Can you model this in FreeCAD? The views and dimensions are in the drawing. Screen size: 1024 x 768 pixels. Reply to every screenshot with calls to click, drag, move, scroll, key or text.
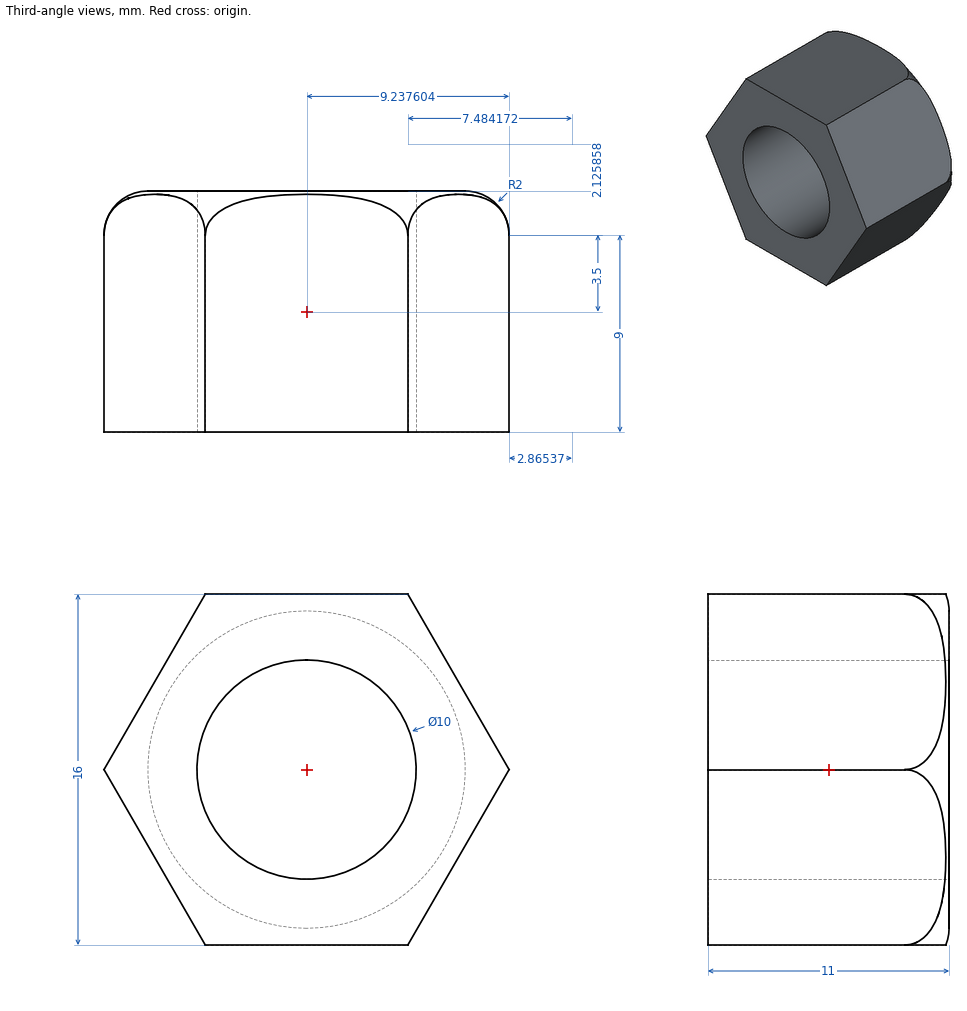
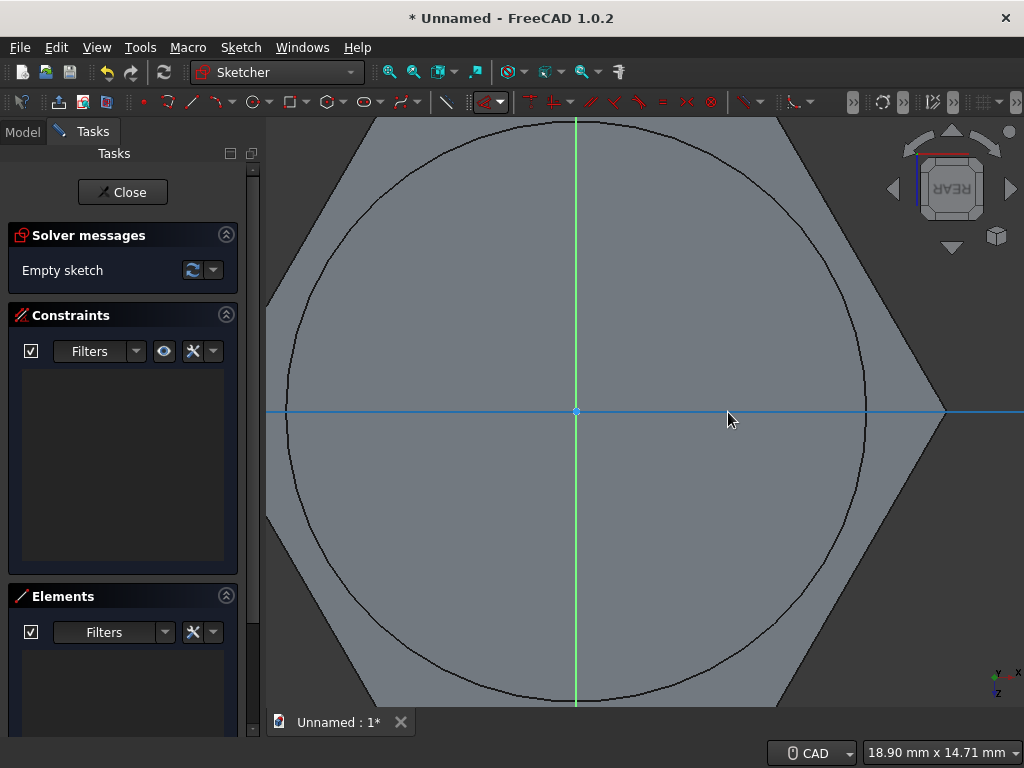
key(g)
key(c)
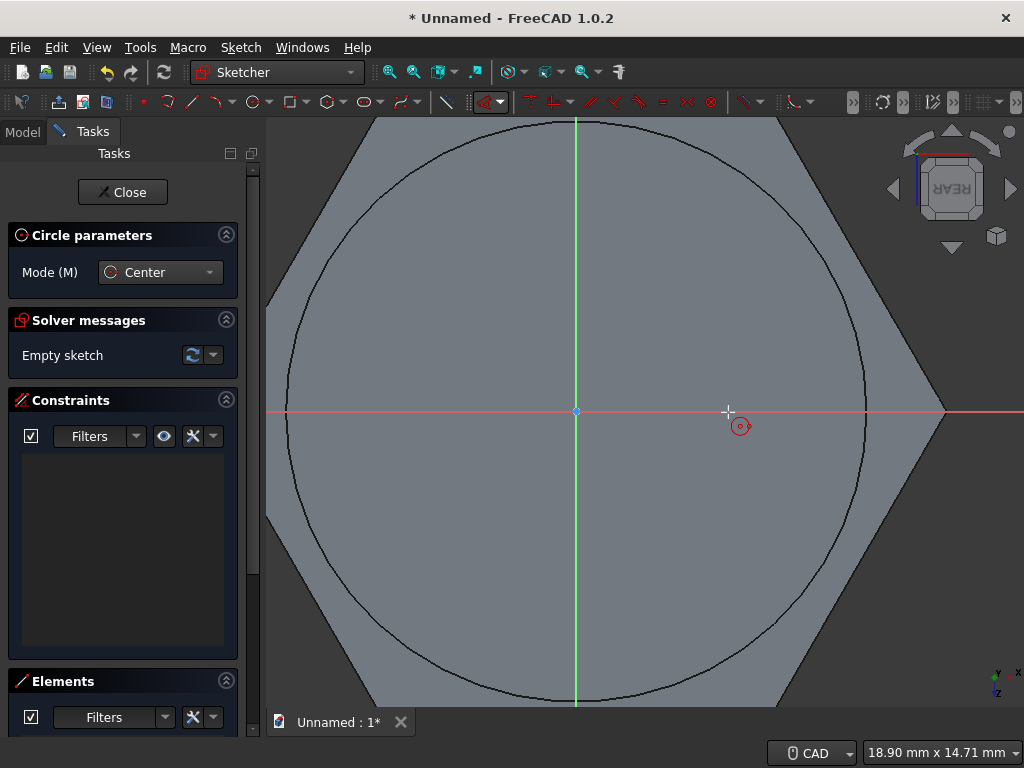
click(576, 412)
click(718, 270)
key(Escape)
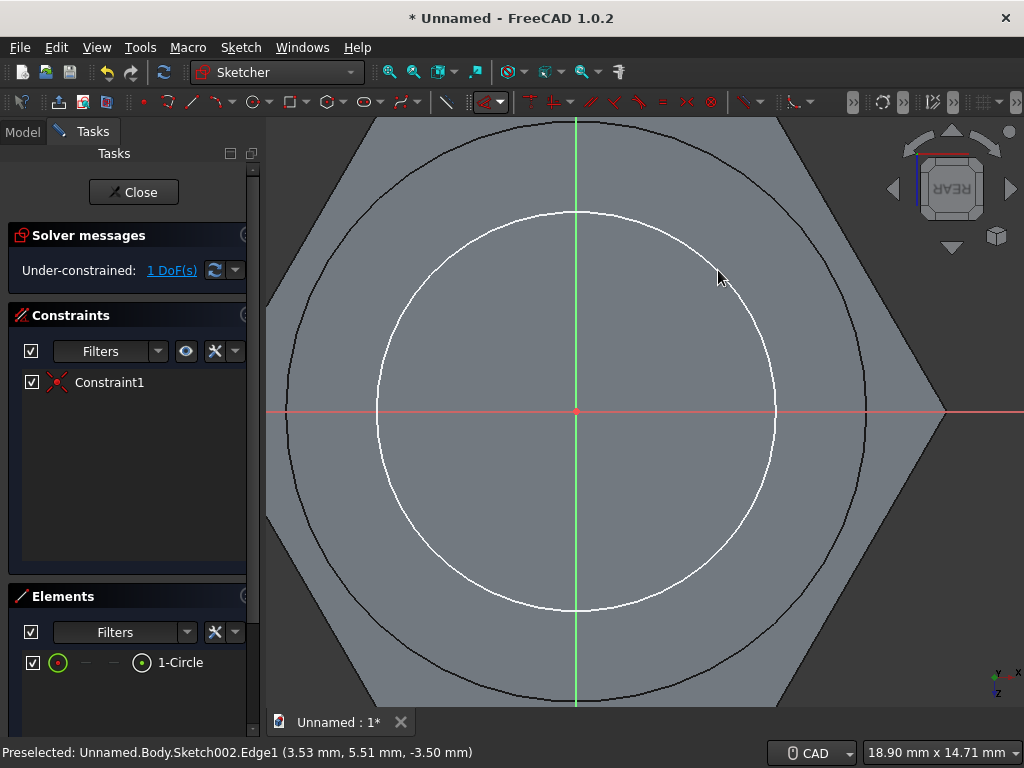
click(717, 270)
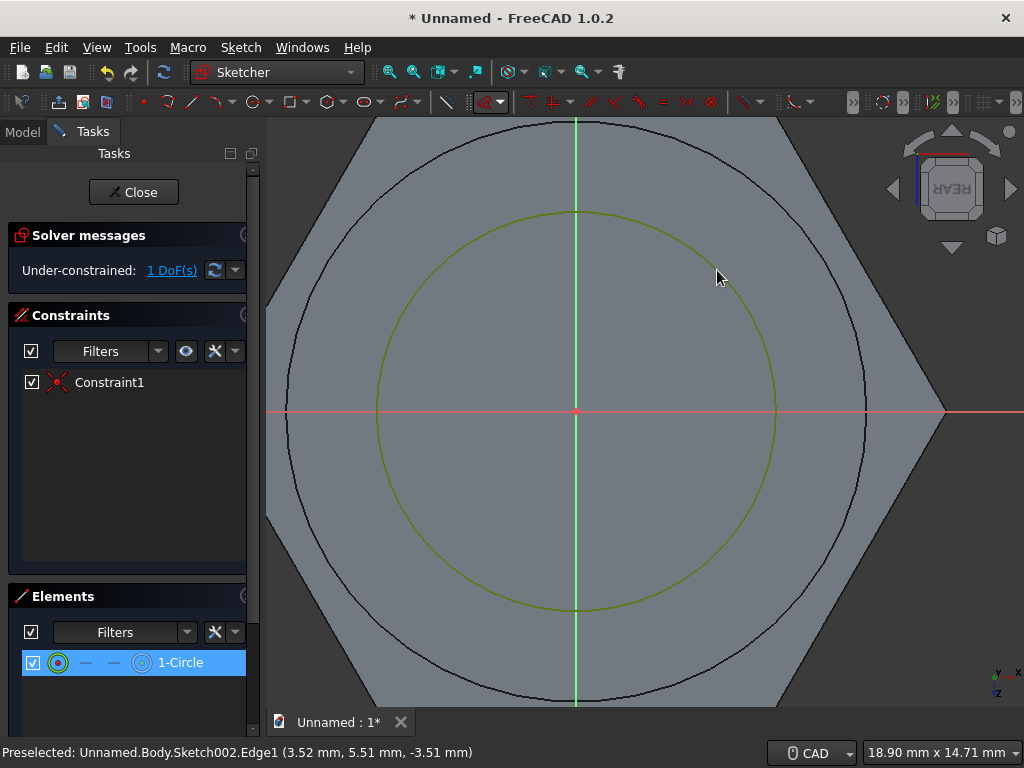
key(k)
key(o)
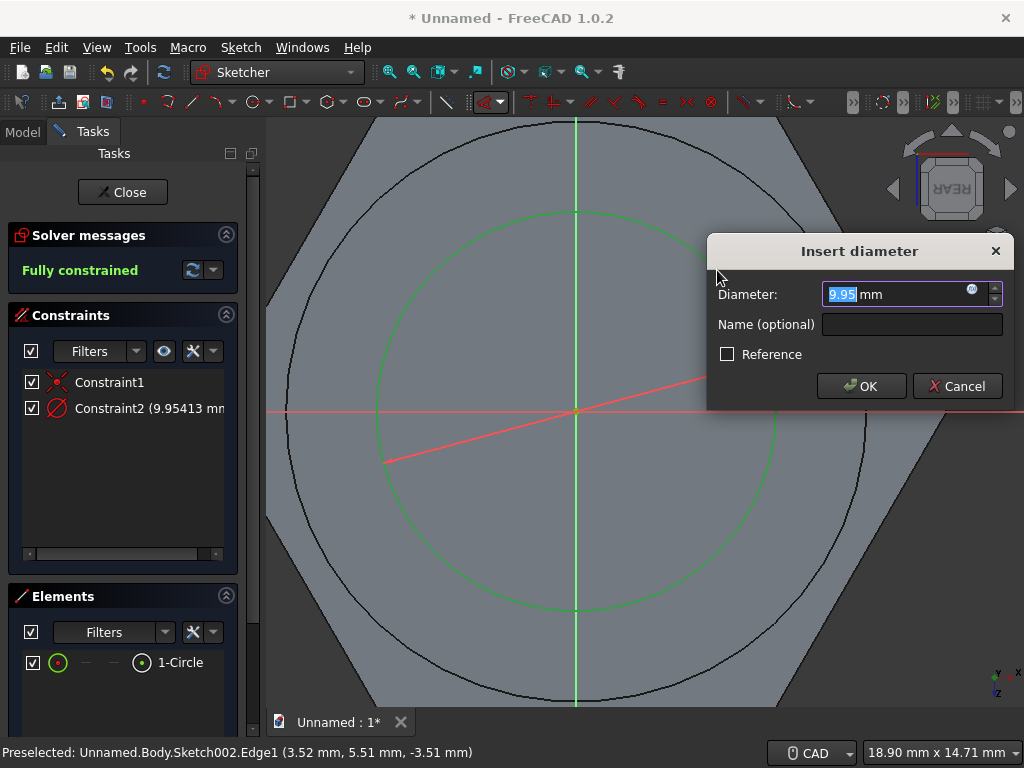
text(10)
key(Return)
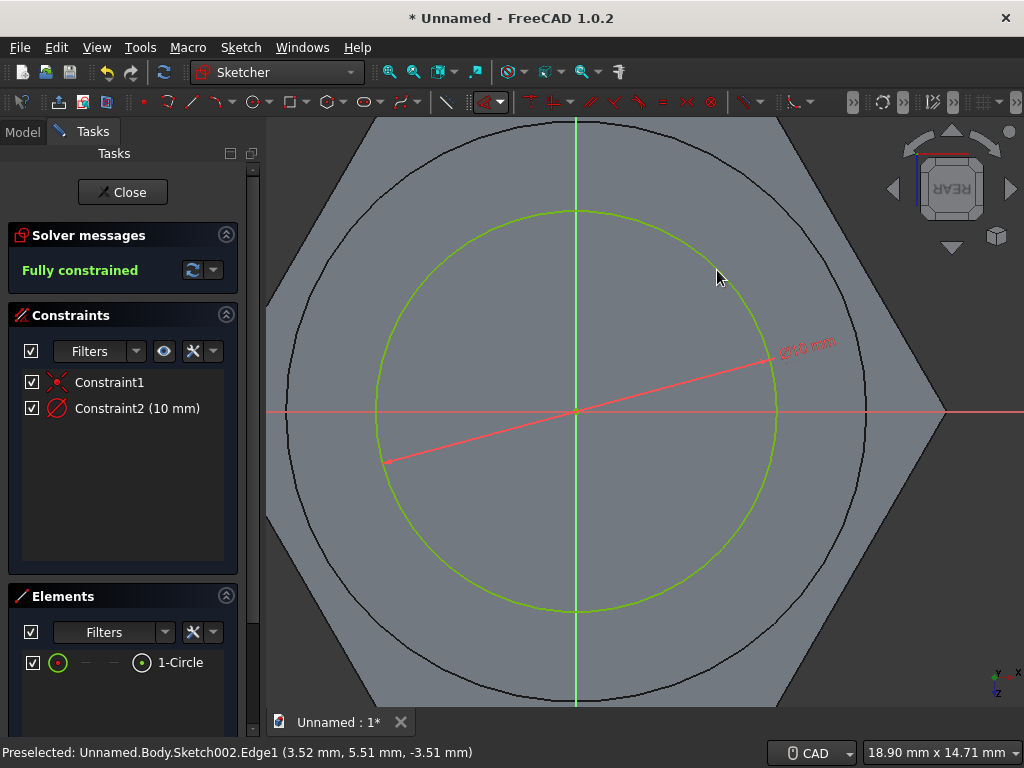
click(123, 192)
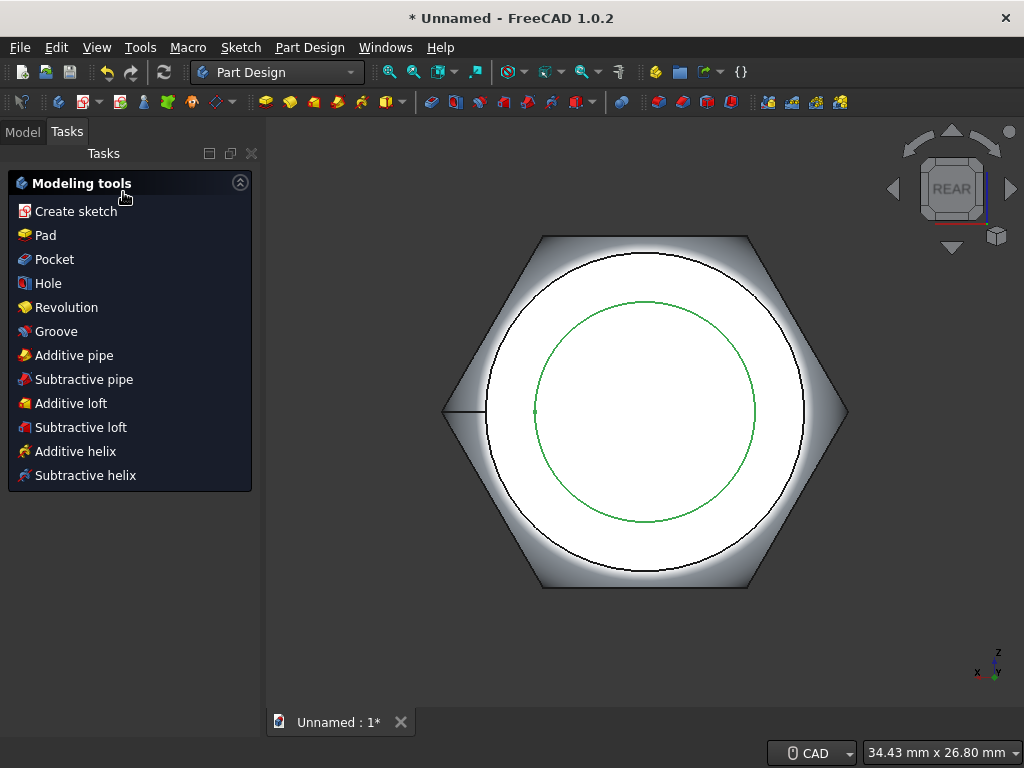
click(432, 102)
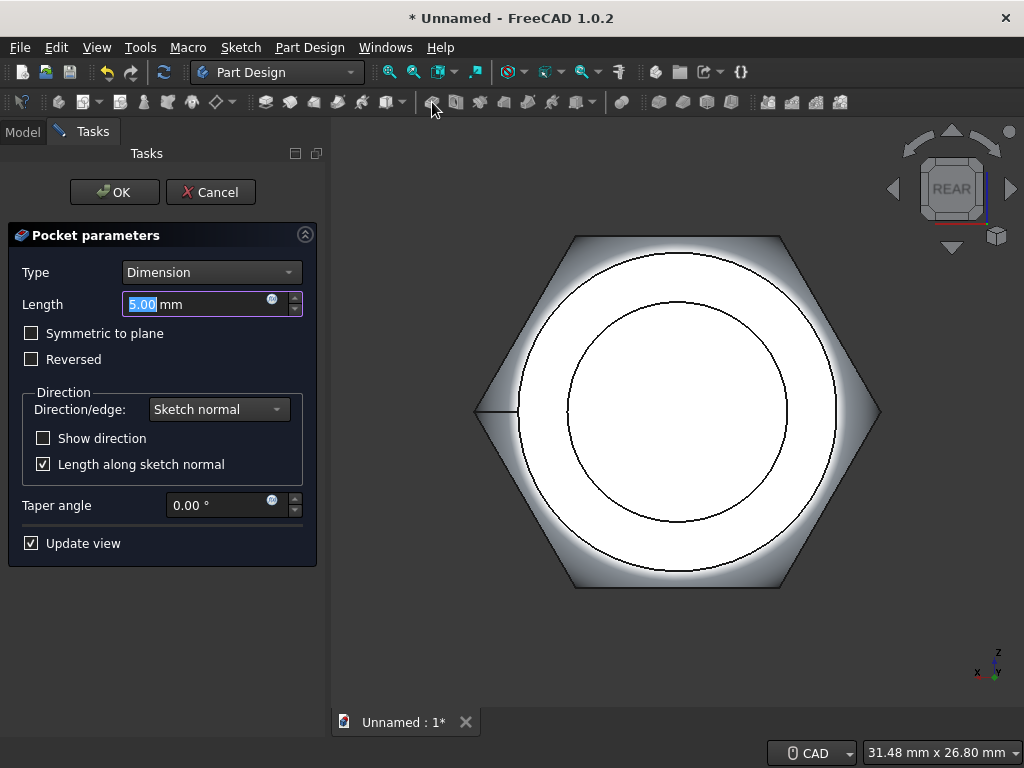
click(212, 272)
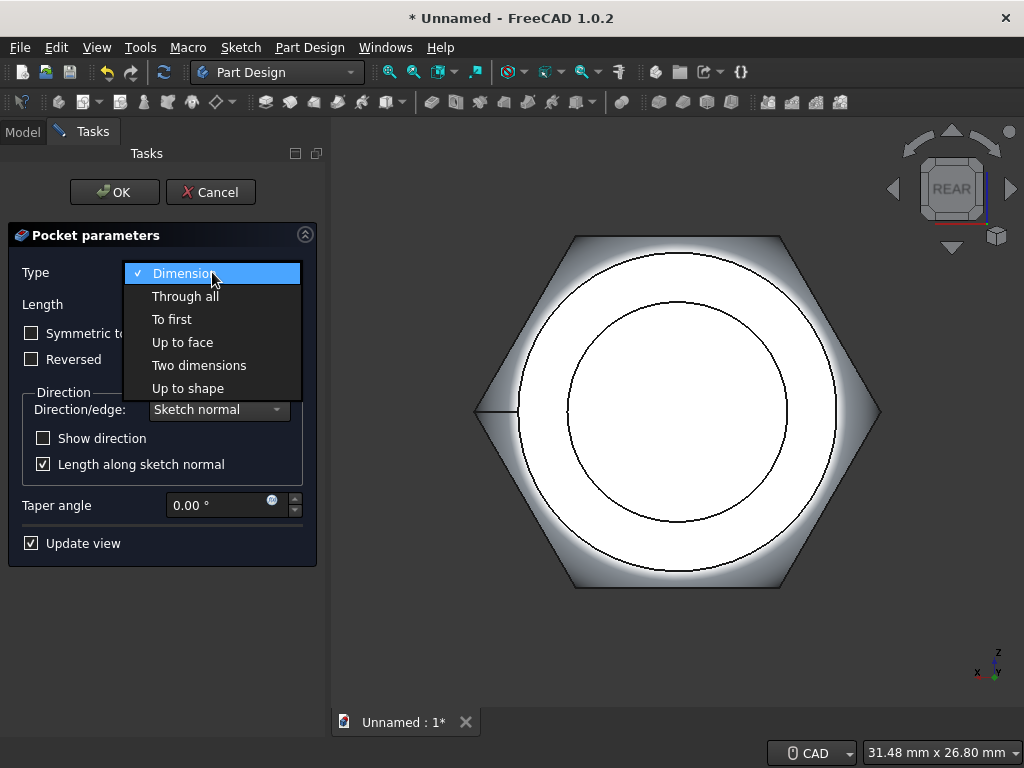
click(212, 296)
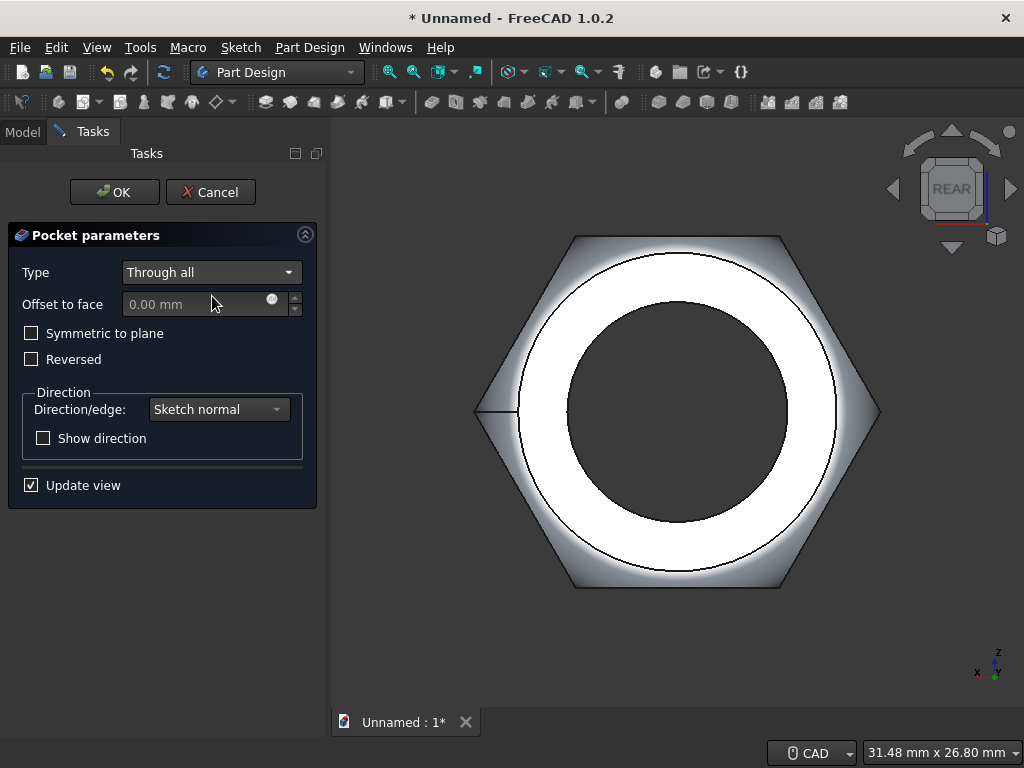
click(115, 192)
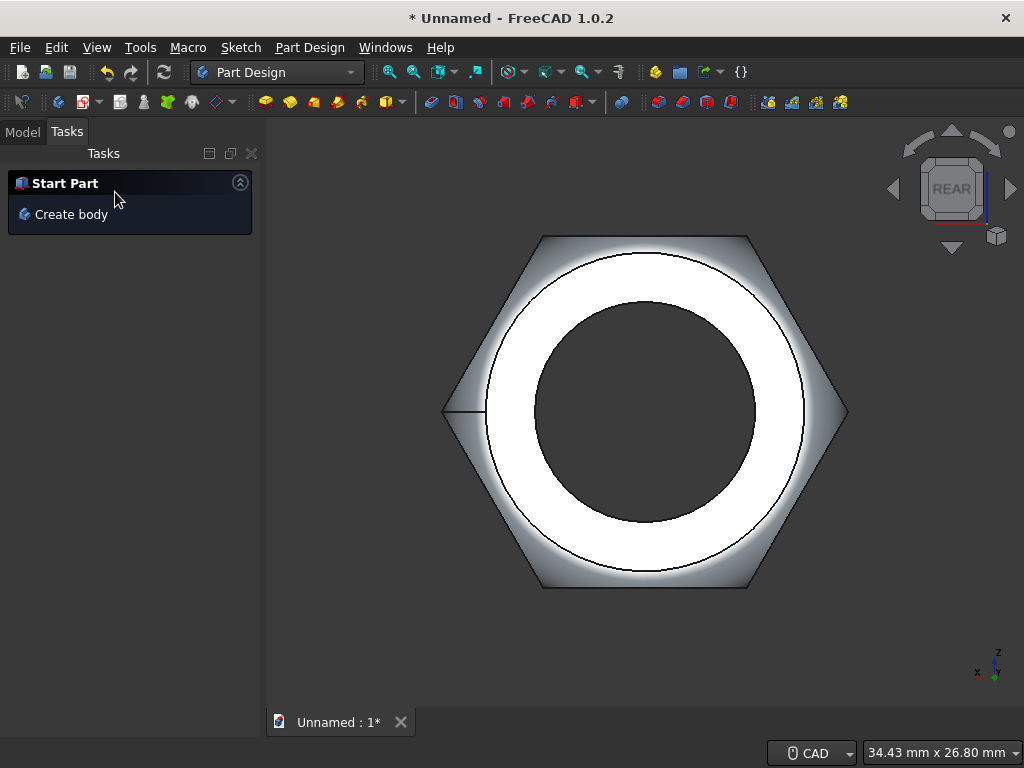
key(0)